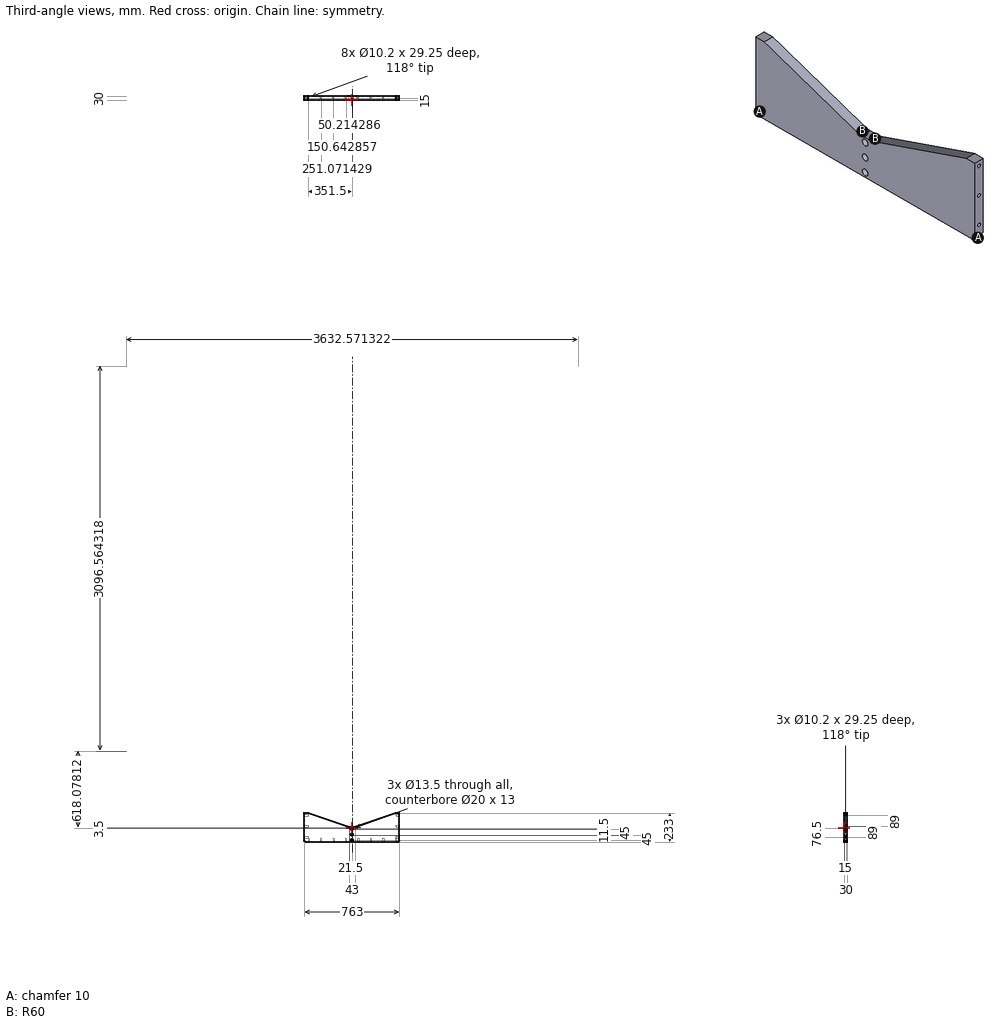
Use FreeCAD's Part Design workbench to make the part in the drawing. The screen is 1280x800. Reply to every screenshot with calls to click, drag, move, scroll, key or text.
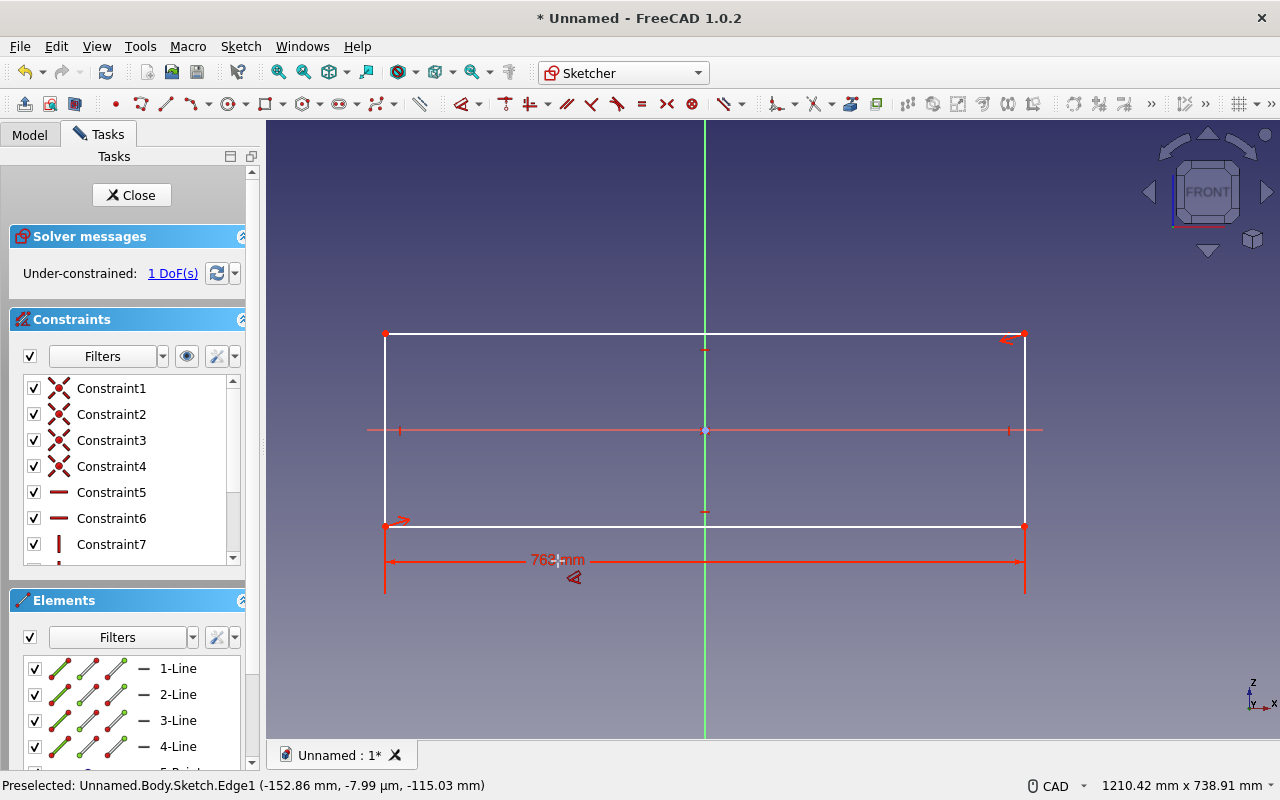
click(1025, 469)
click(1059, 386)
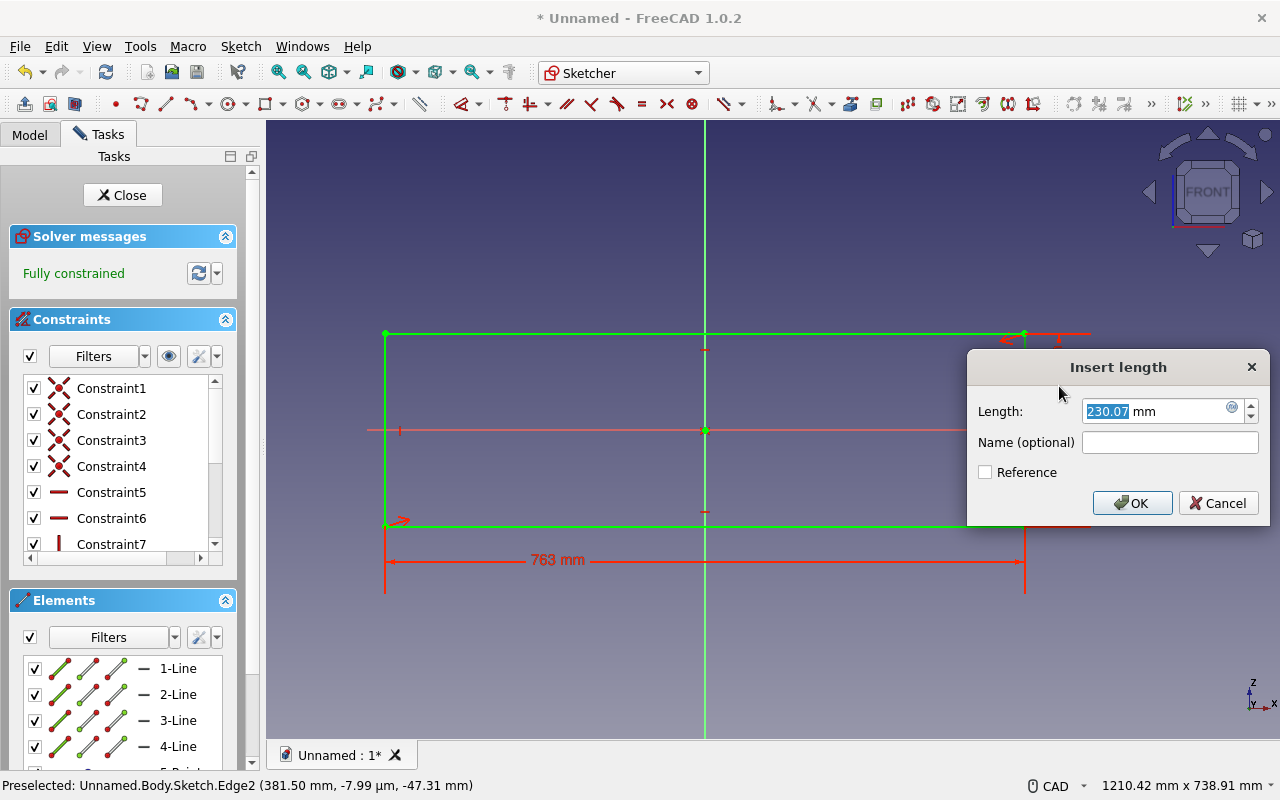
text(233)
key(Return)
key(Escape)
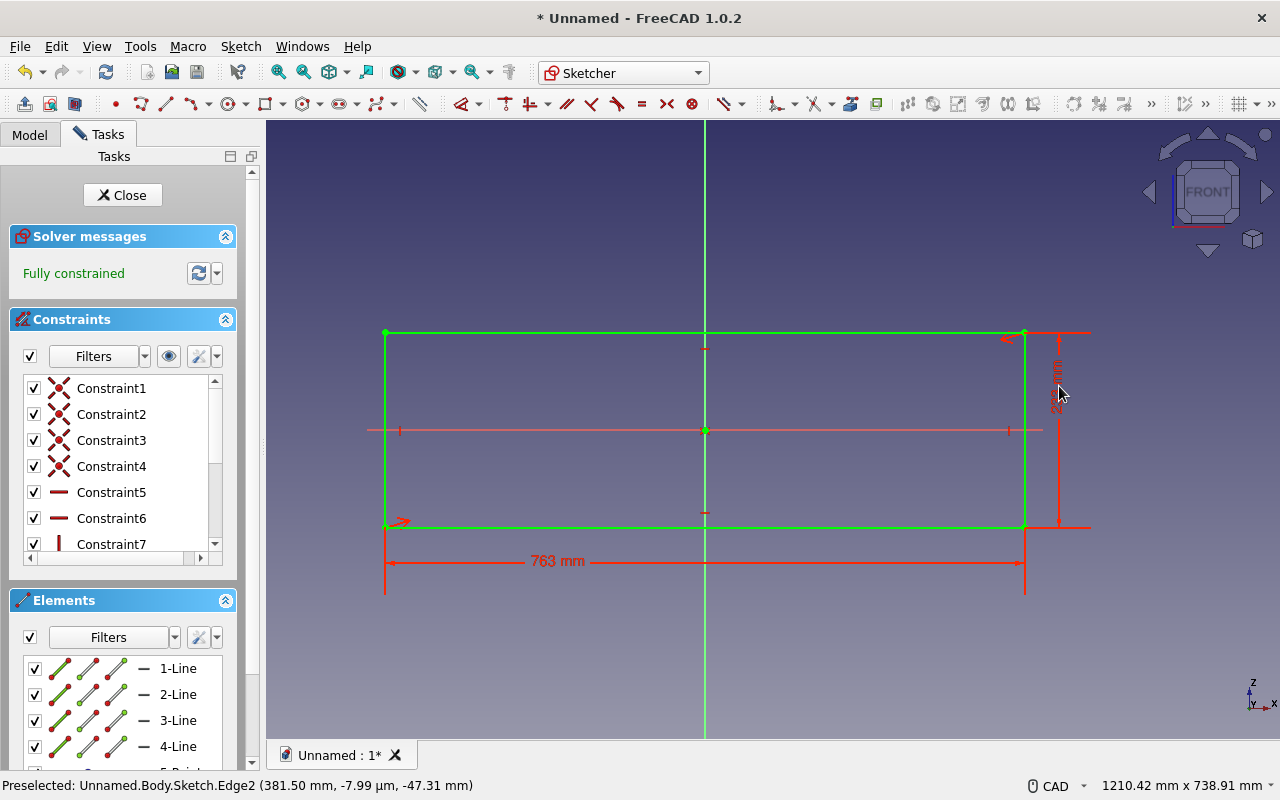
click(123, 195)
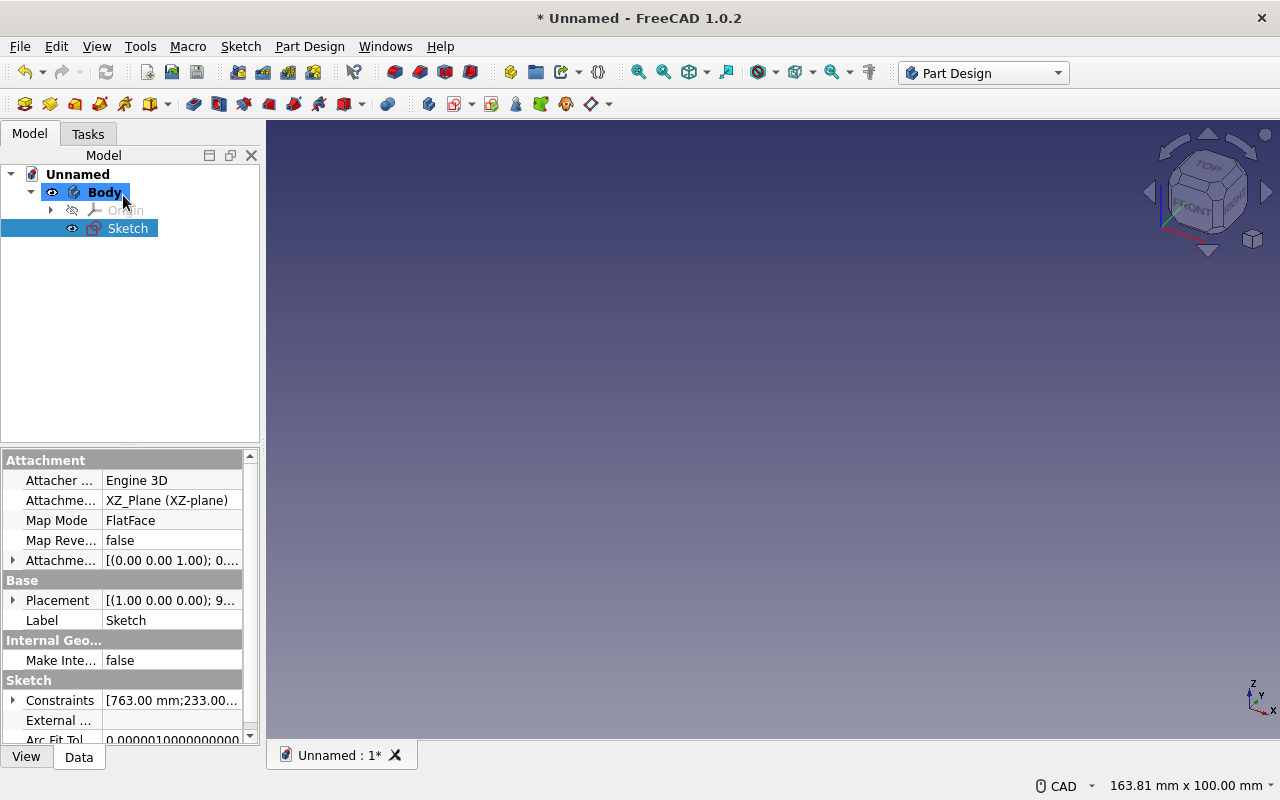
click(25, 104)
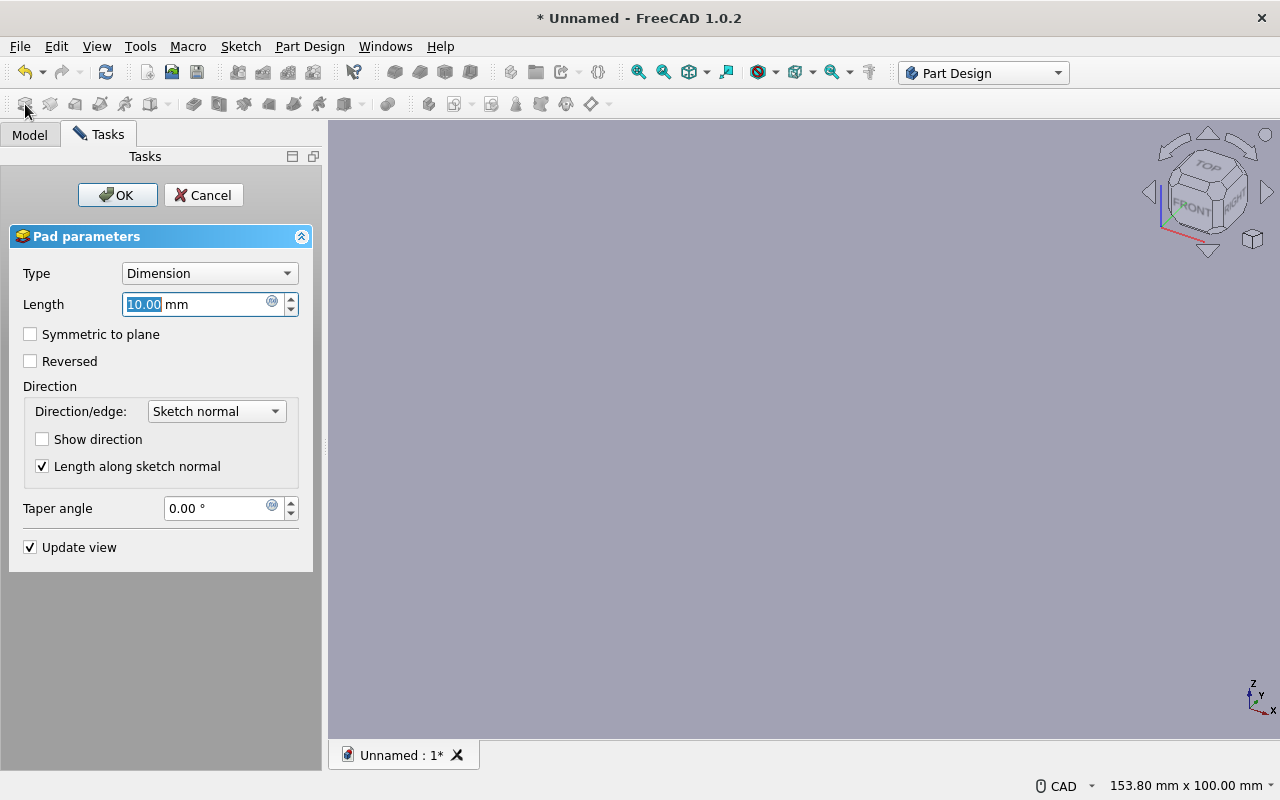
text(30)
key(Tab)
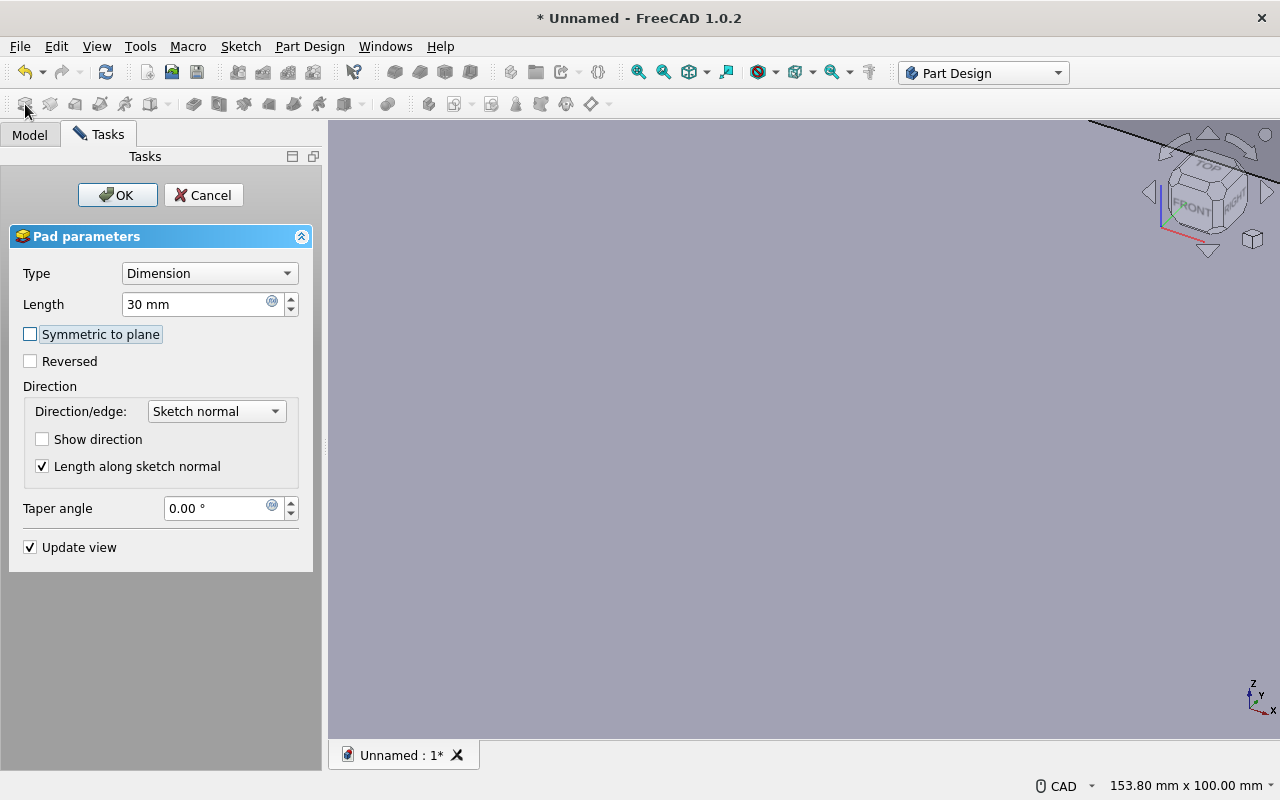
click(31, 361)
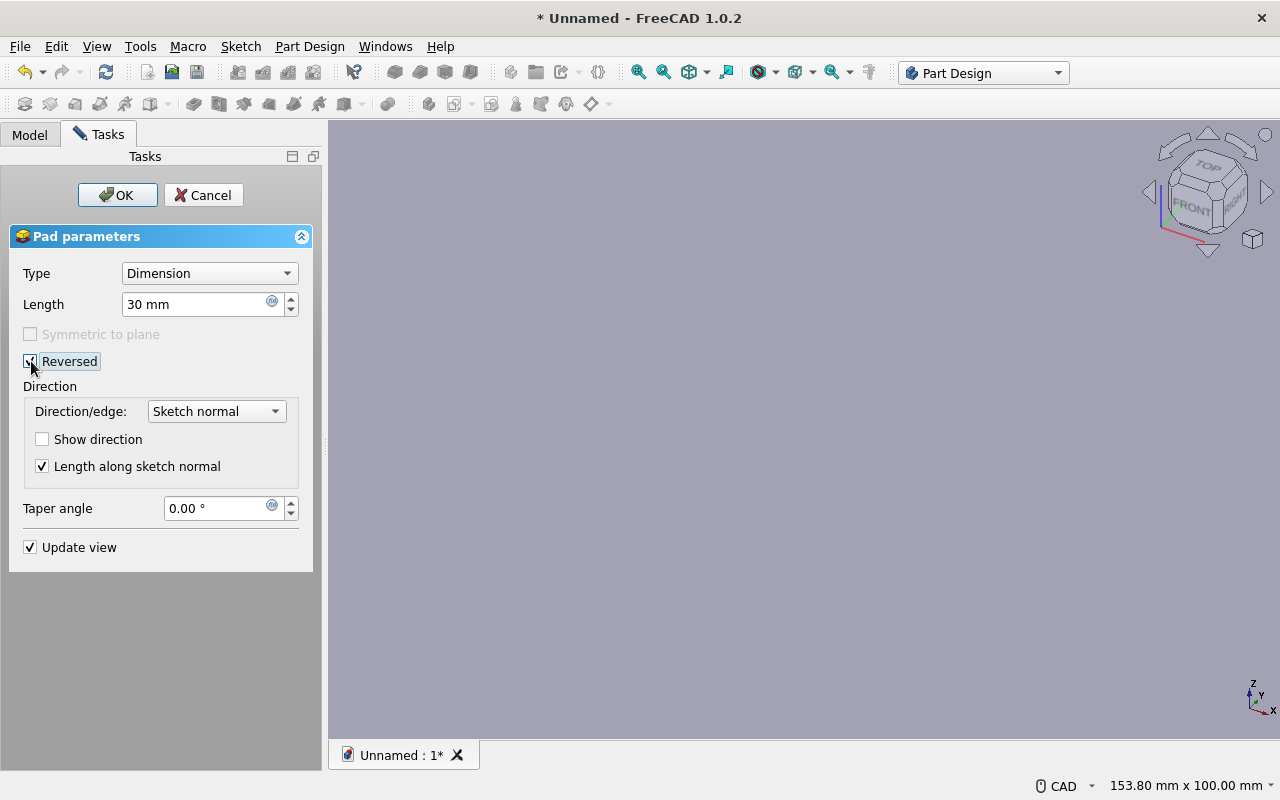
click(118, 195)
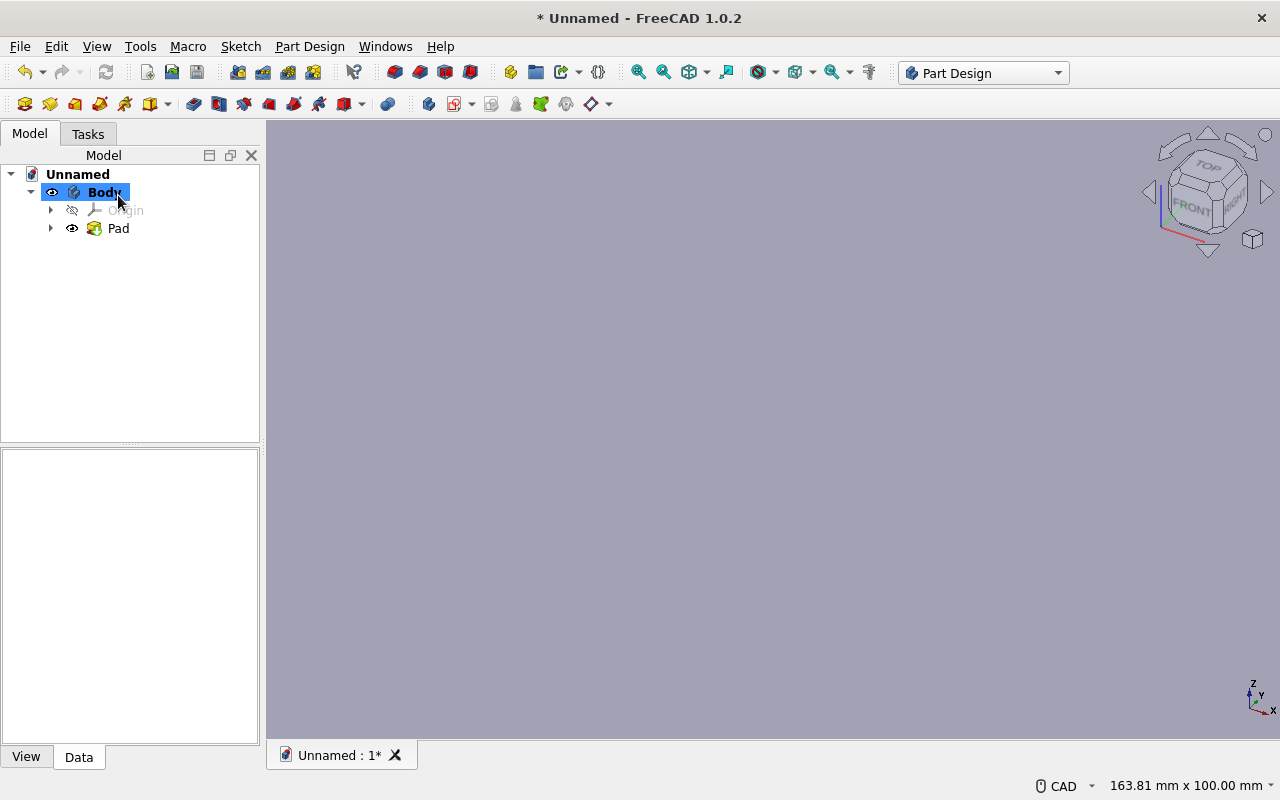
click(639, 72)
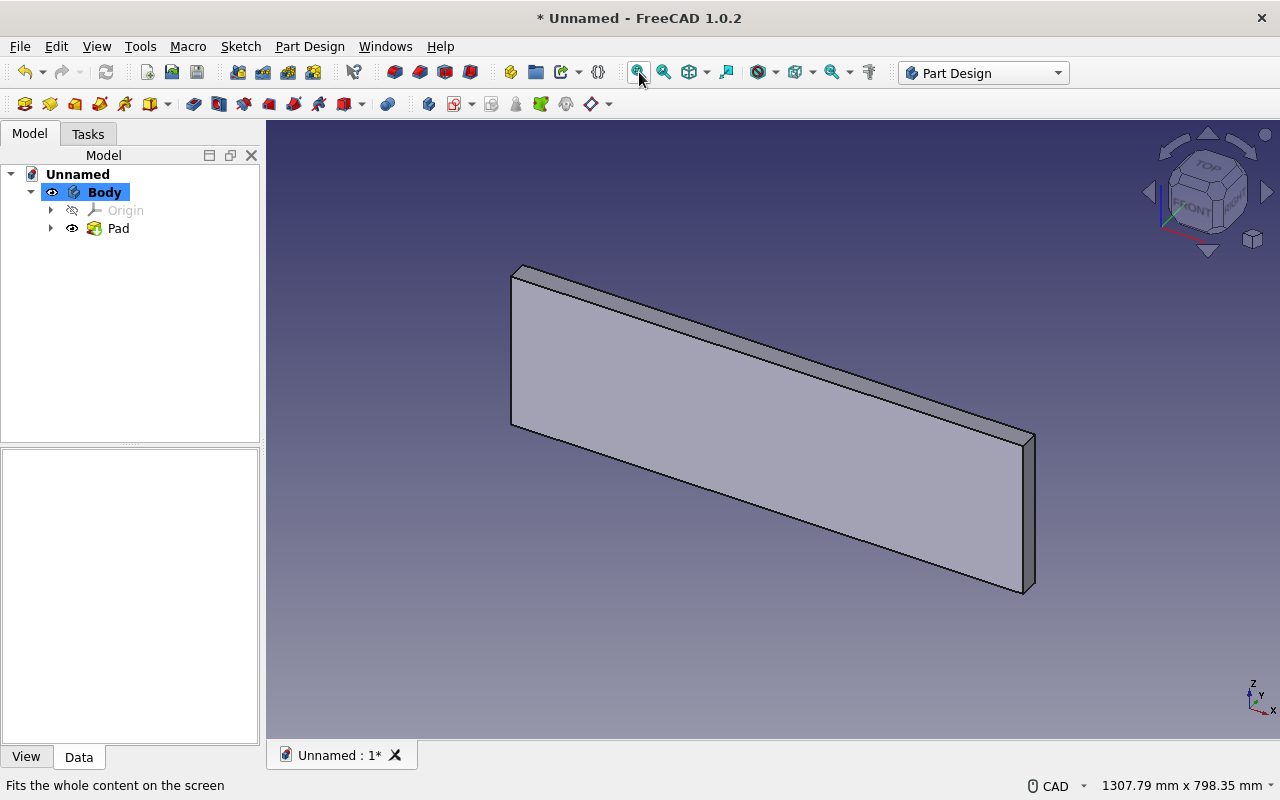
key(0)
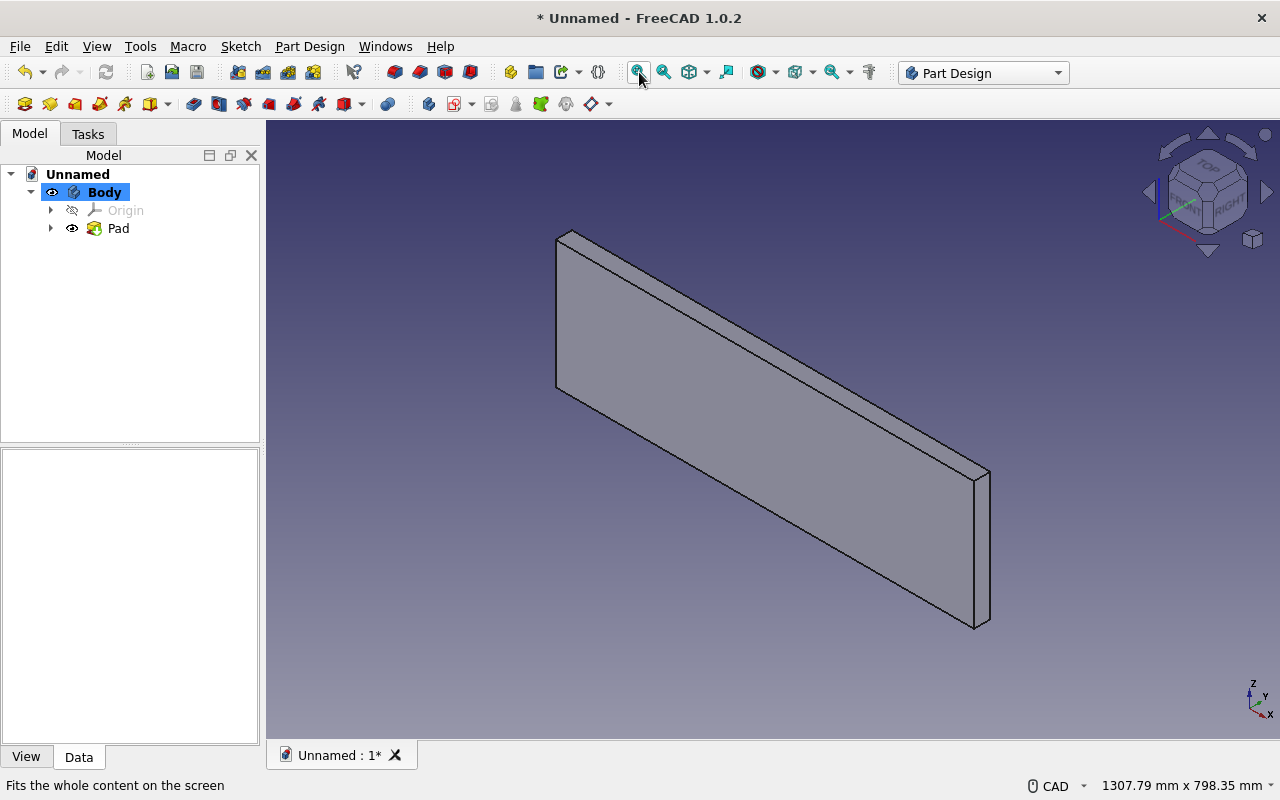
key(2)